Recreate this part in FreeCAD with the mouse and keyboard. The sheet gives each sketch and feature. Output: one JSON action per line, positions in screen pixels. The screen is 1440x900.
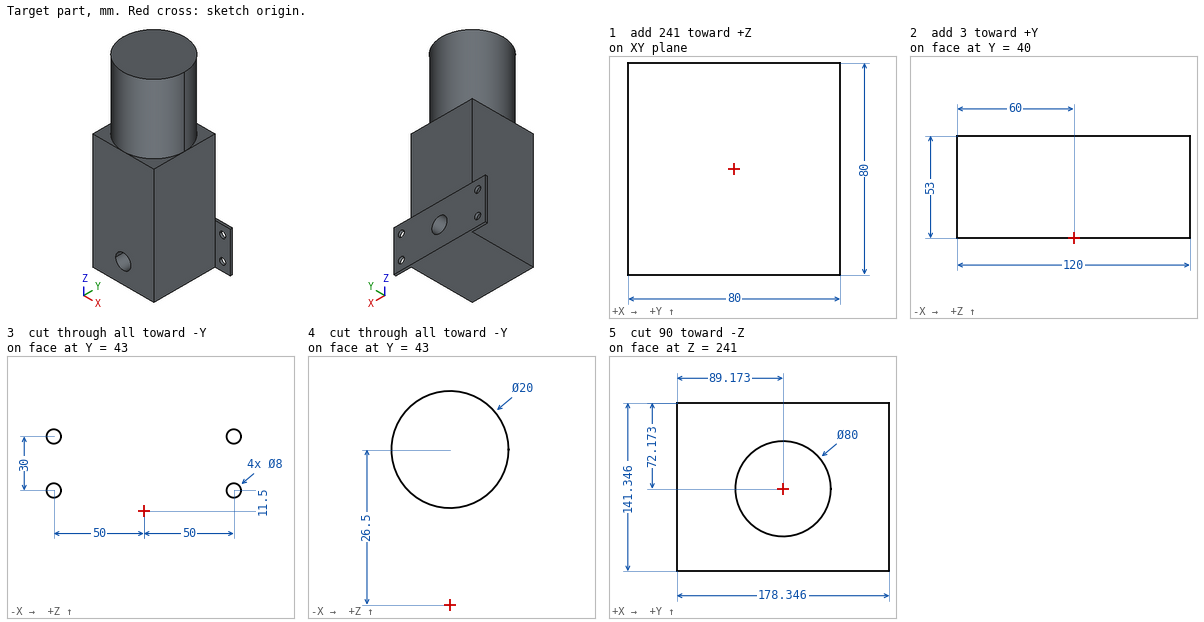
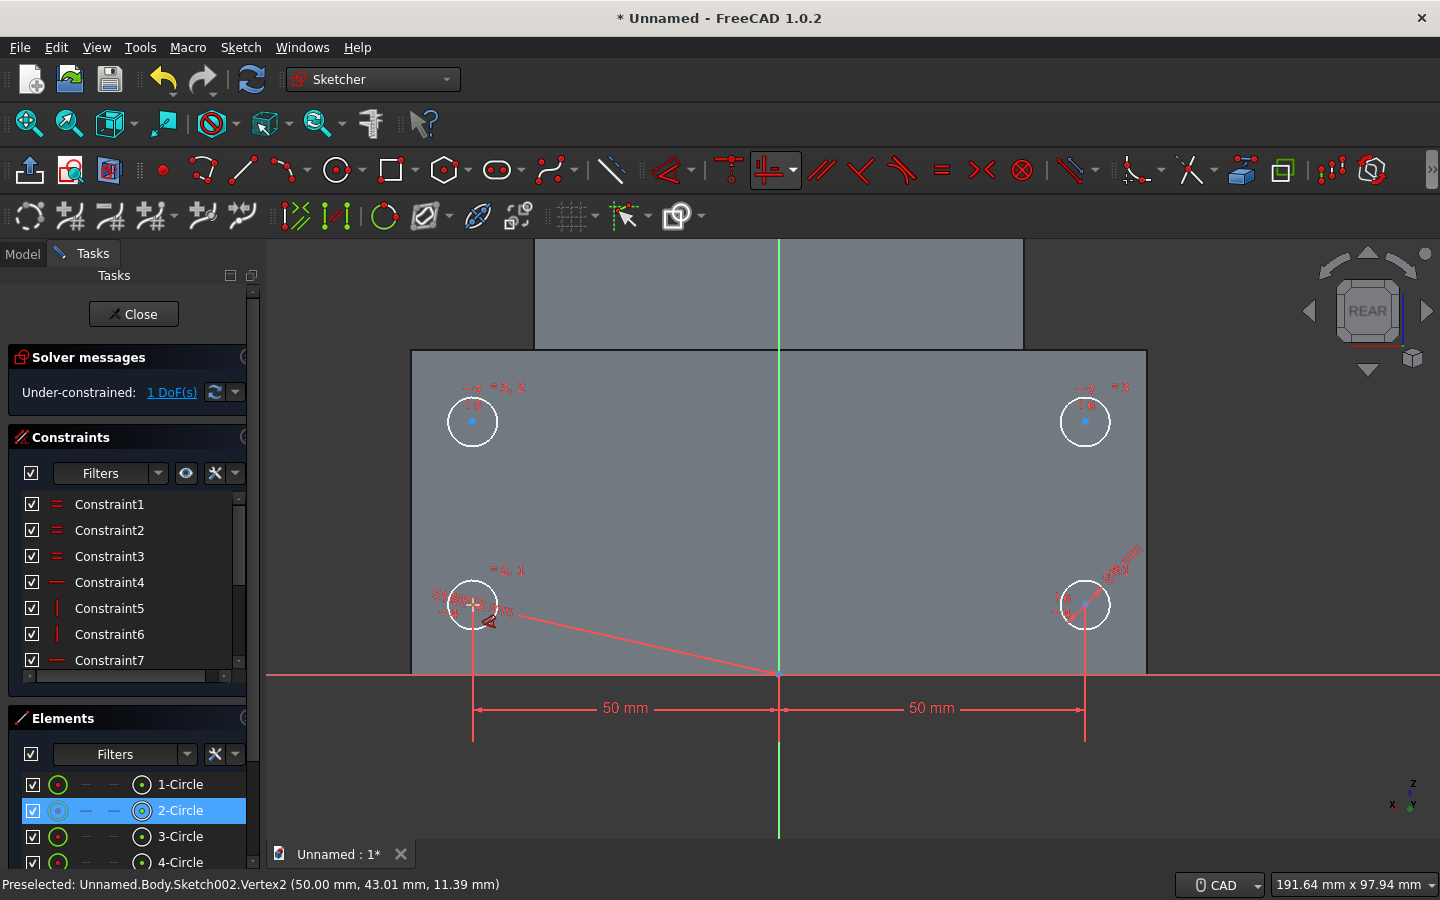
{"action": "left_click", "coordinate": [473, 422]}
{"action": "left_click", "coordinate": [439, 514]}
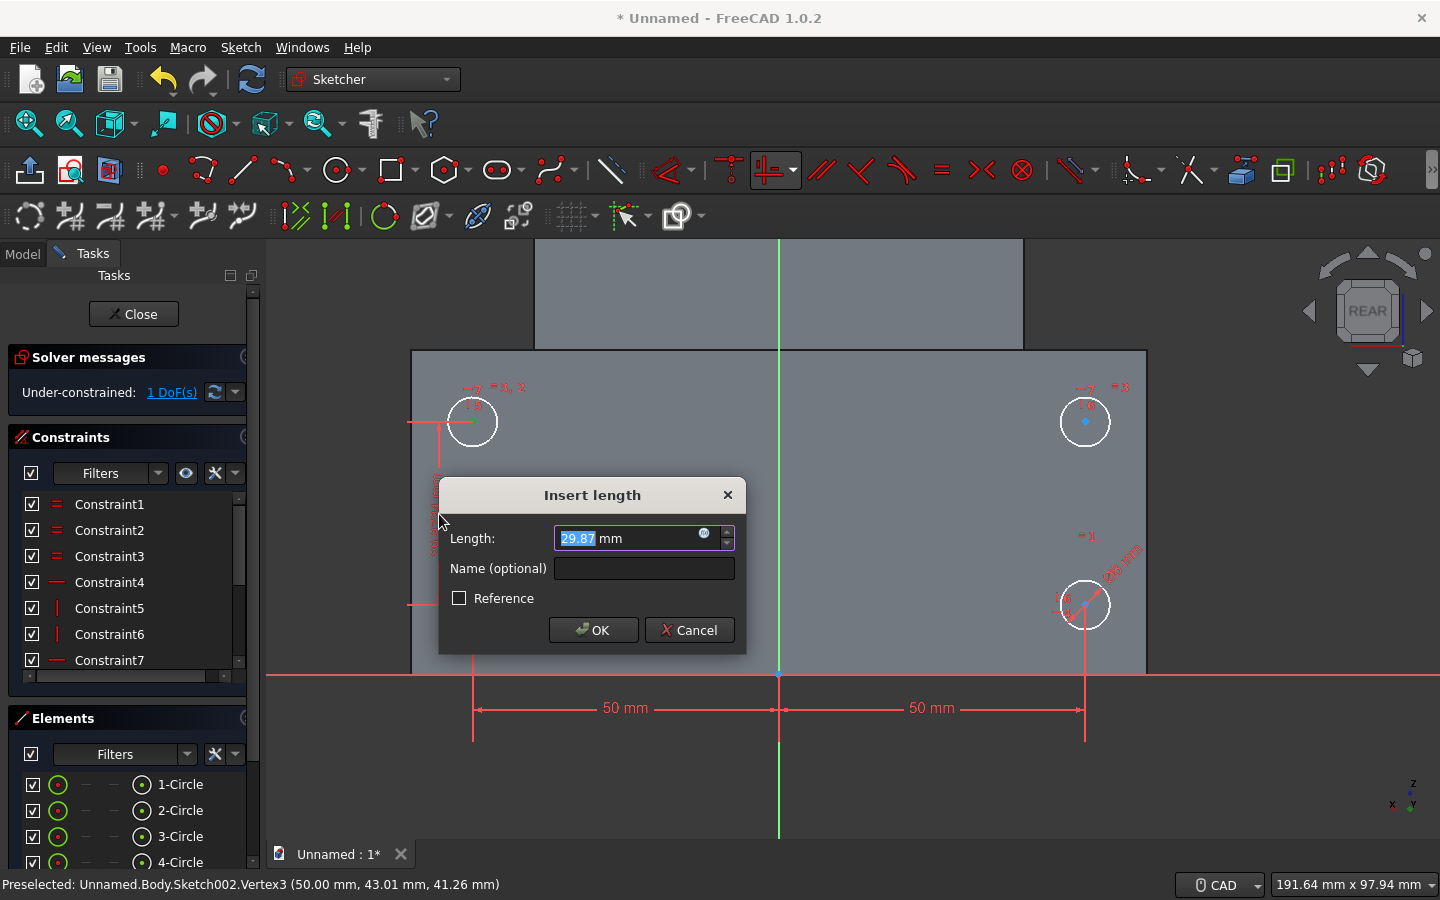
{"action": "type", "text": "30"}
{"action": "key", "text": "Return"}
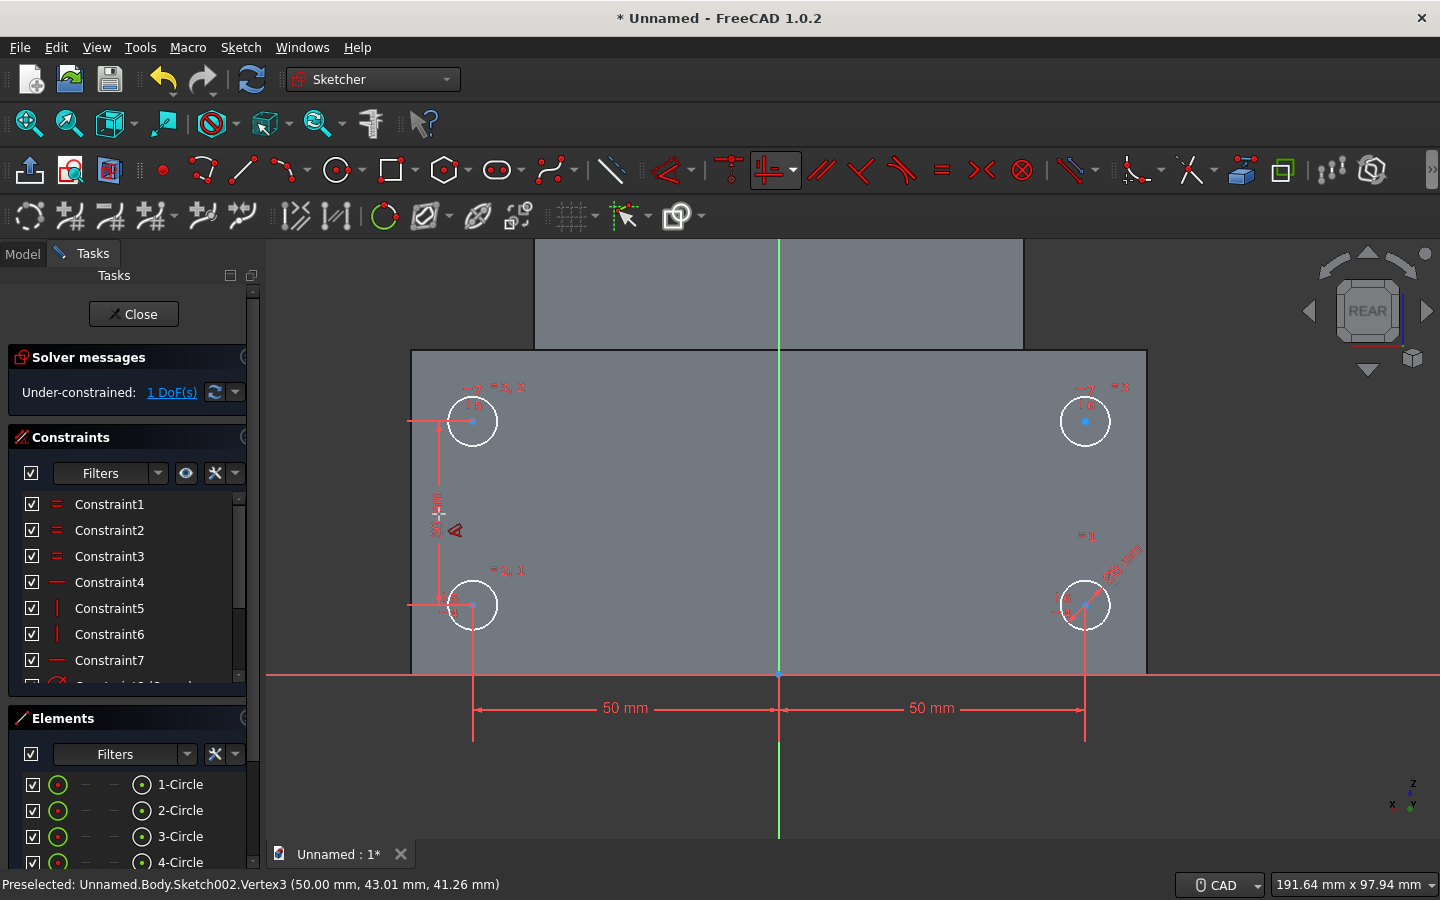
{"action": "left_click", "coordinate": [1085, 605]}
{"action": "left_click", "coordinate": [1119, 640]}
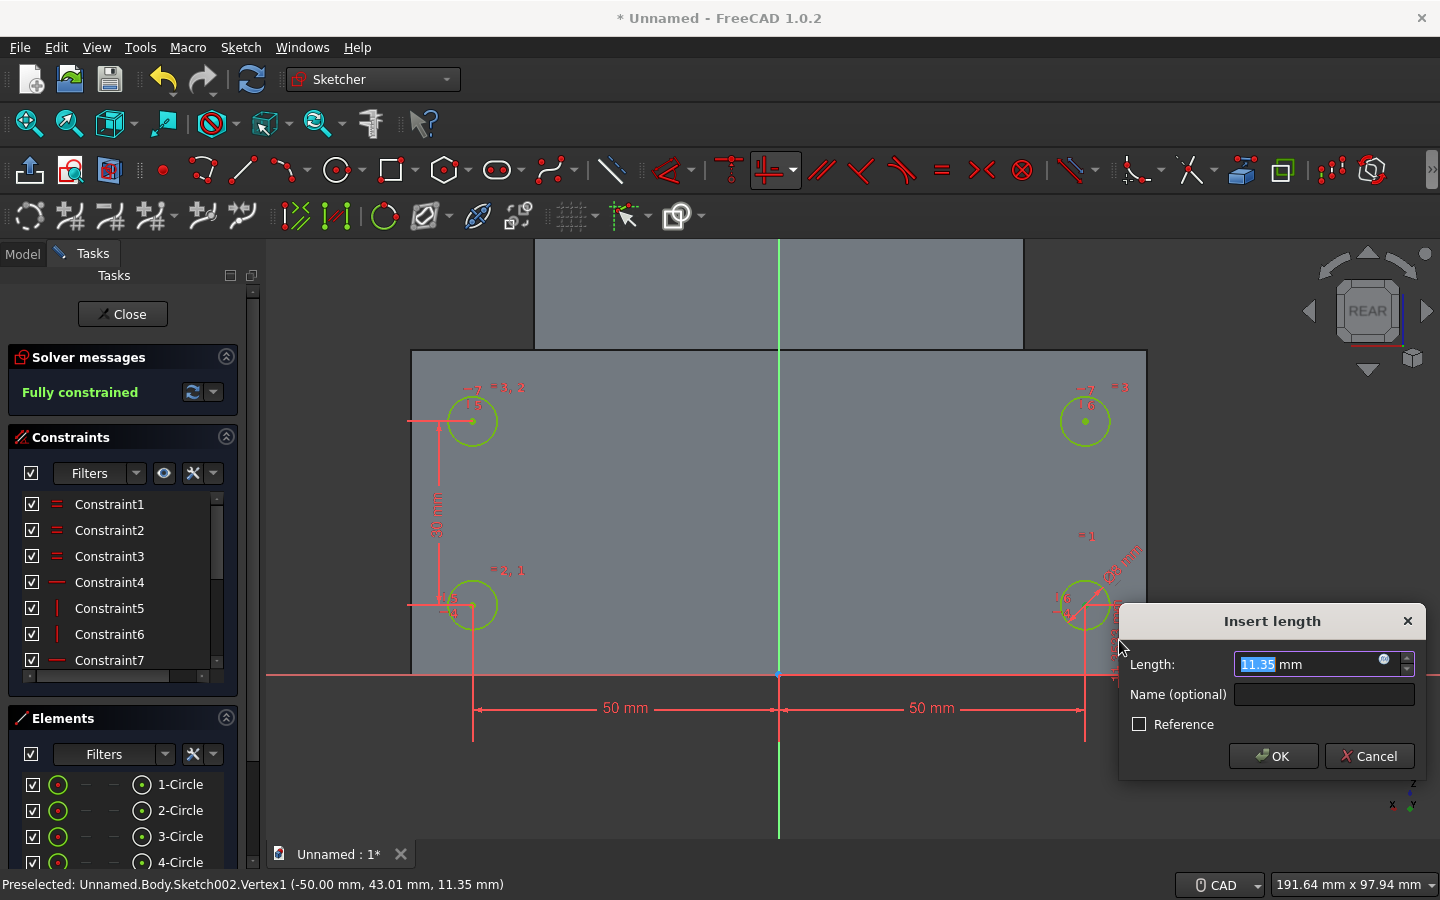
{"action": "type", "text": "11.5"}
{"action": "key", "text": "Return"}
{"action": "key", "text": "Escape"}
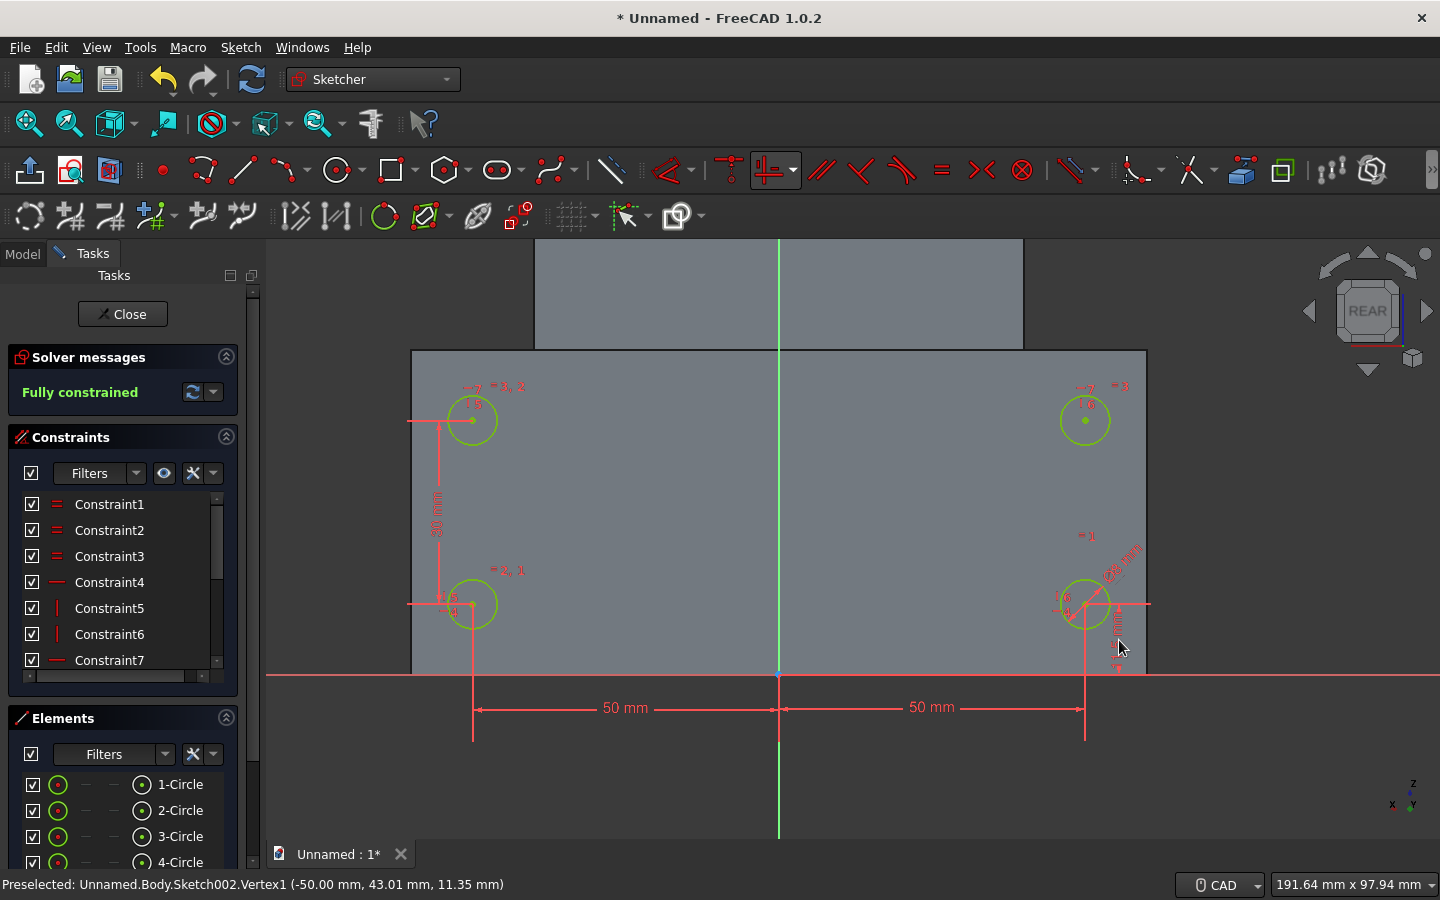
{"action": "left_click", "coordinate": [123, 314]}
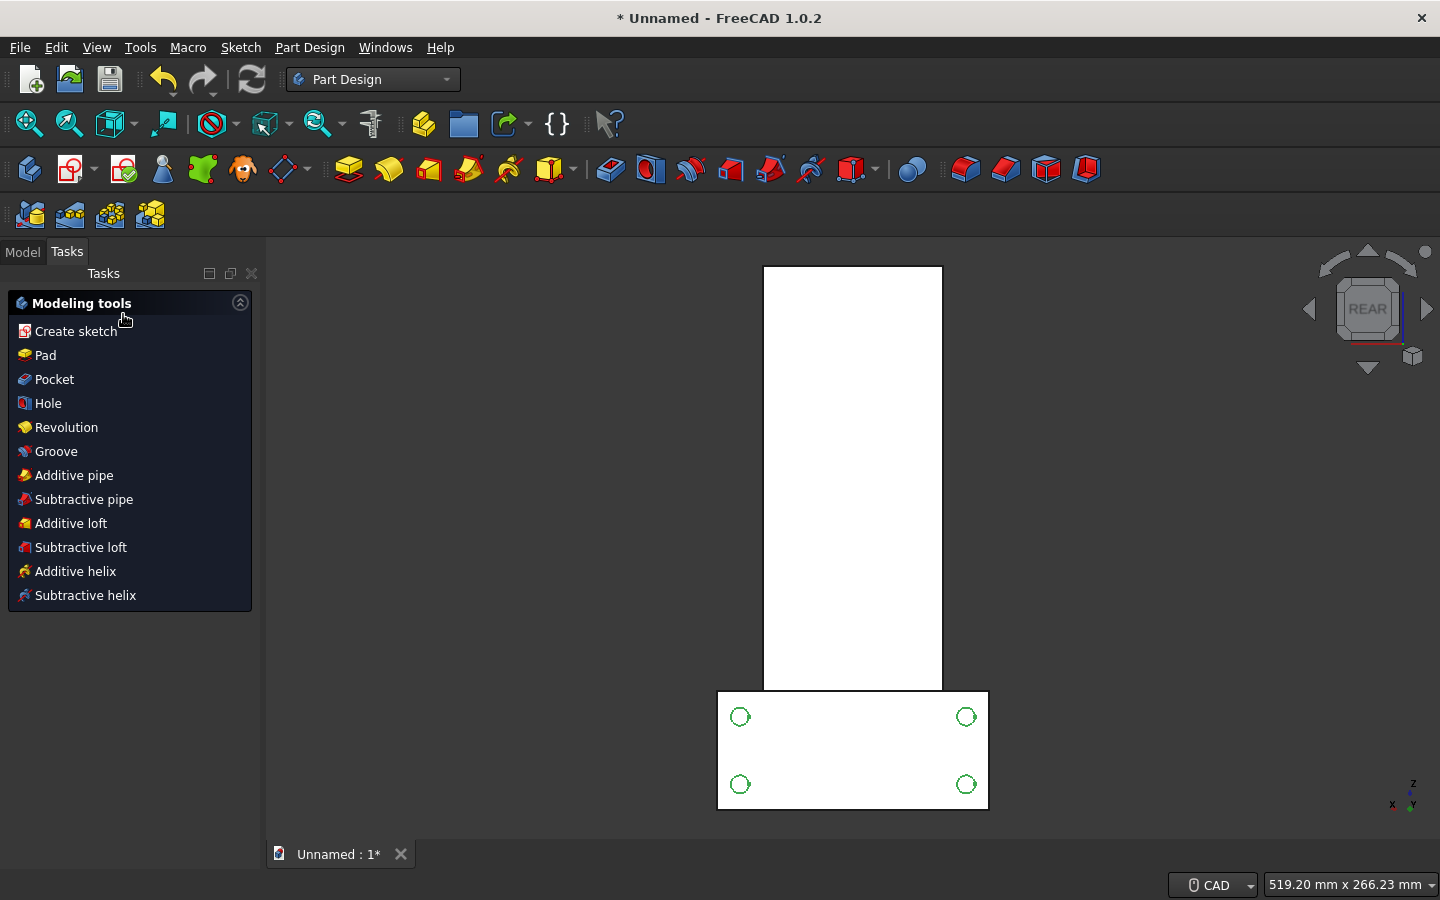
{"action": "left_click", "coordinate": [612, 170]}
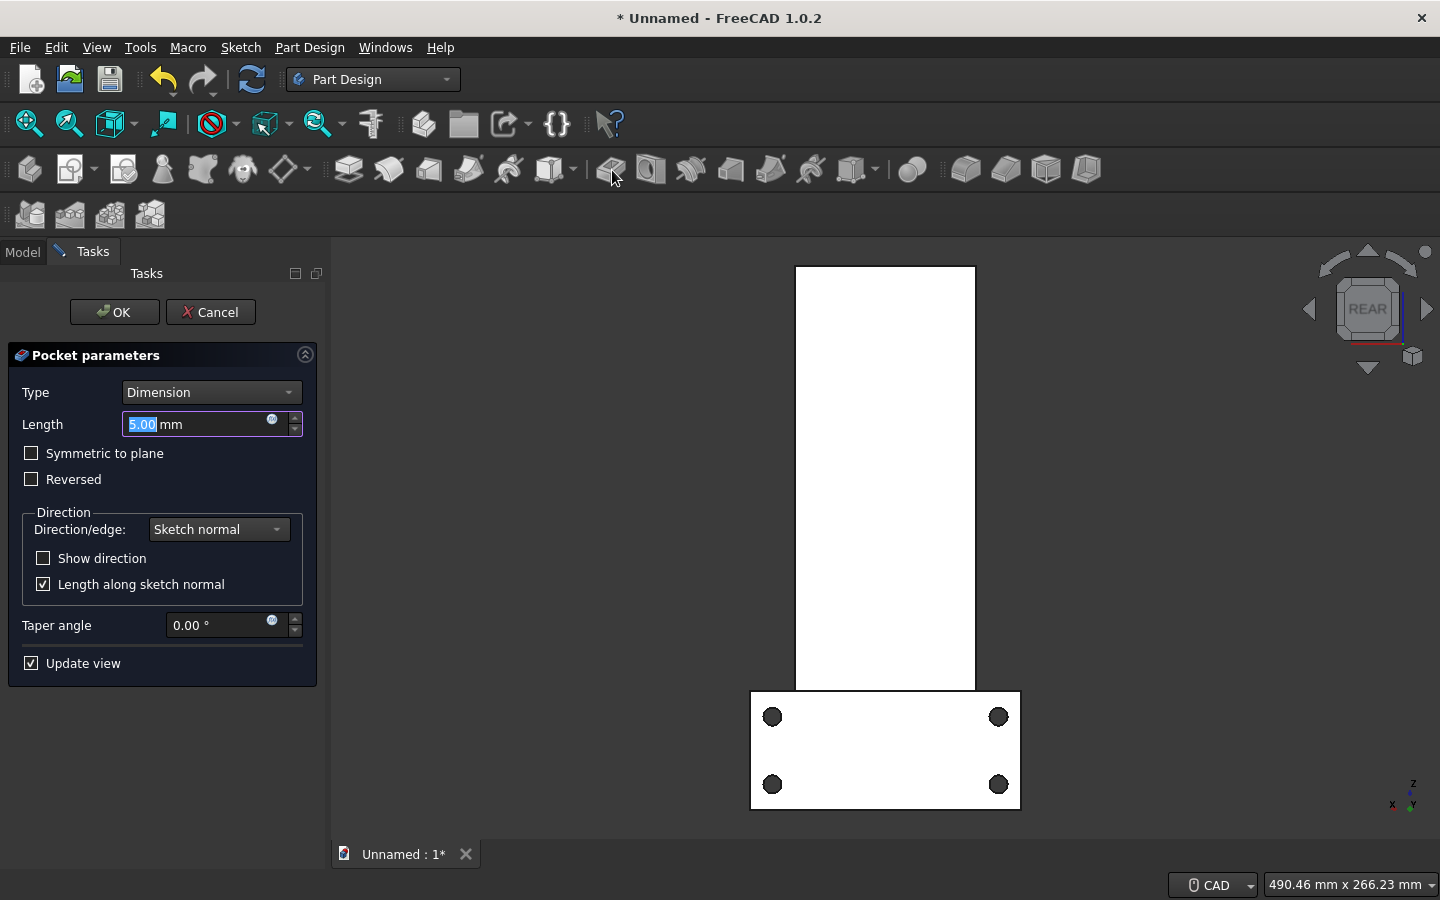
{"action": "left_click", "coordinate": [212, 392]}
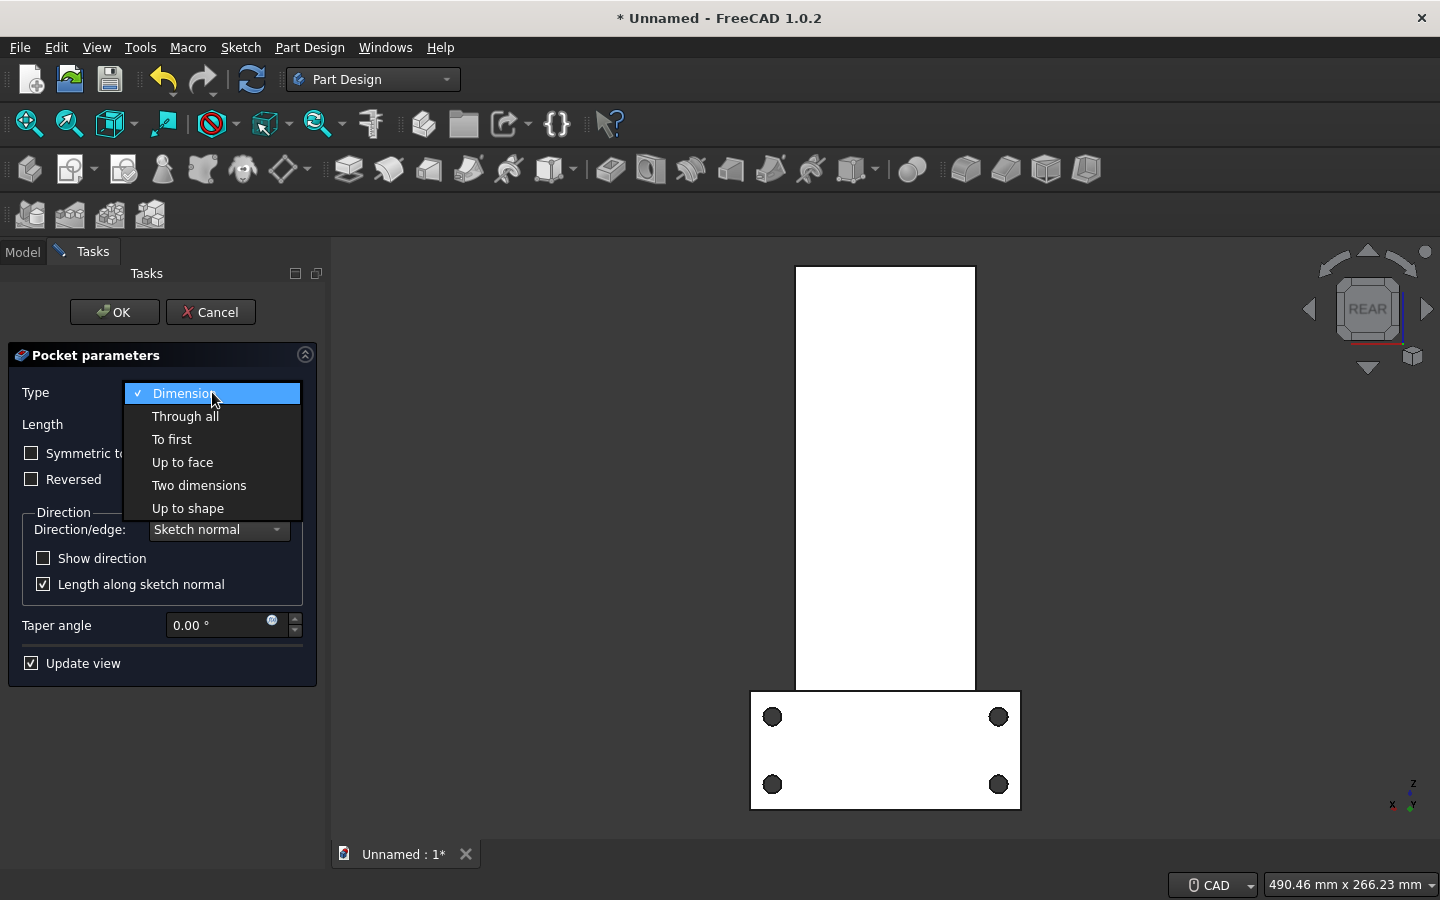
{"action": "left_click", "coordinate": [212, 416]}